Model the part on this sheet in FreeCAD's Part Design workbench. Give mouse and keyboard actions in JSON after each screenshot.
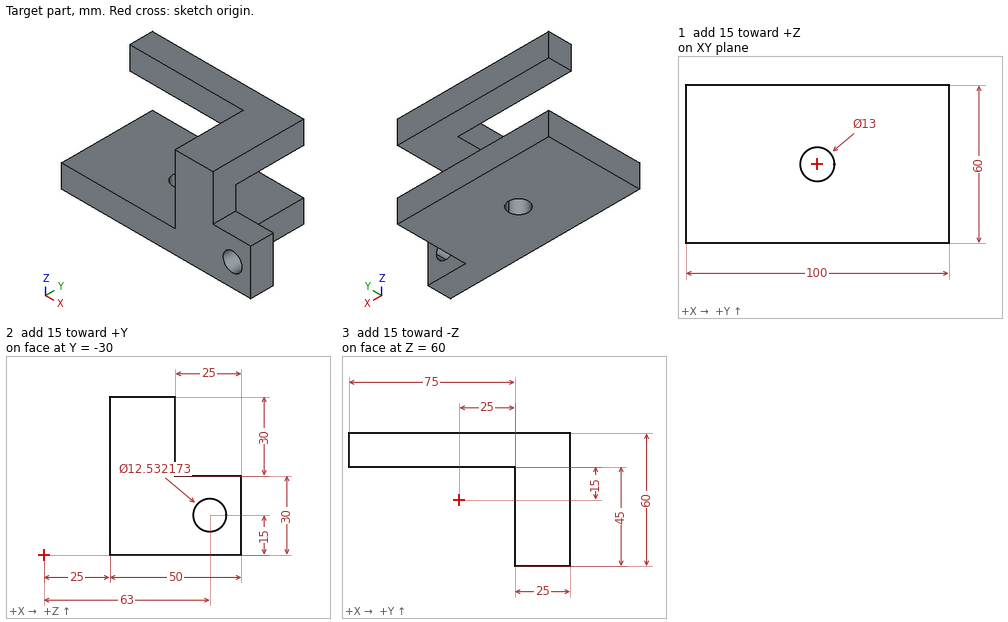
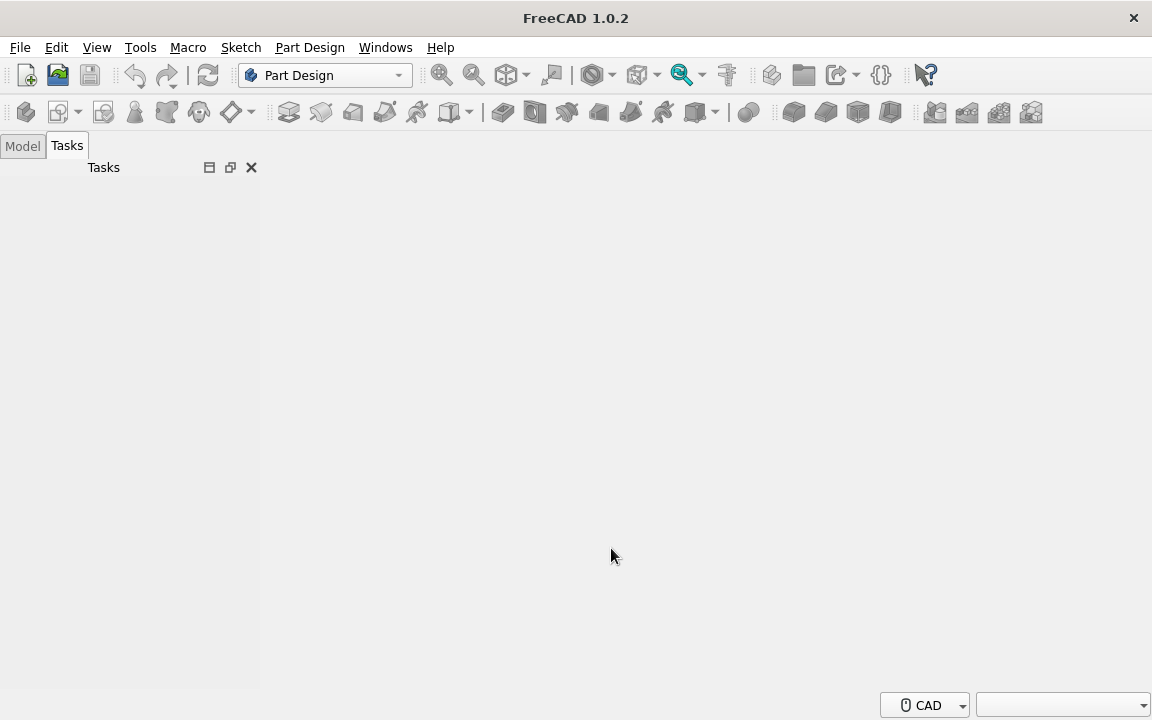
{"action": "key", "text": "ctrl+n"}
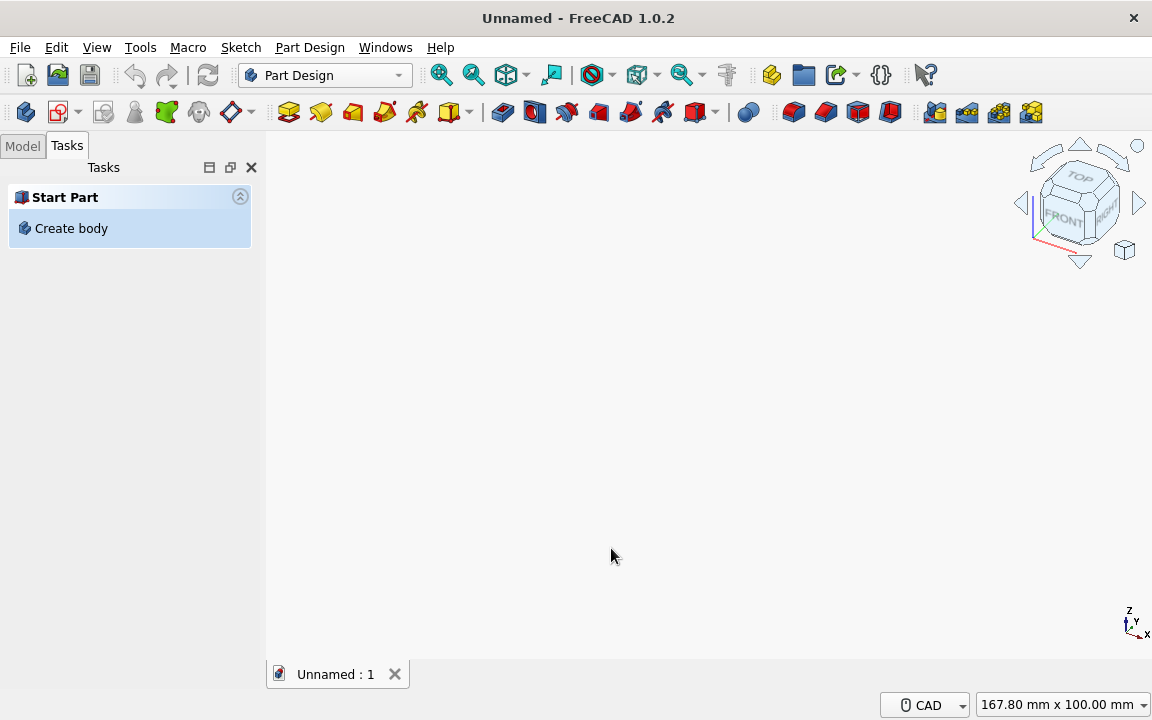
{"action": "left_click", "coordinate": [58, 112]}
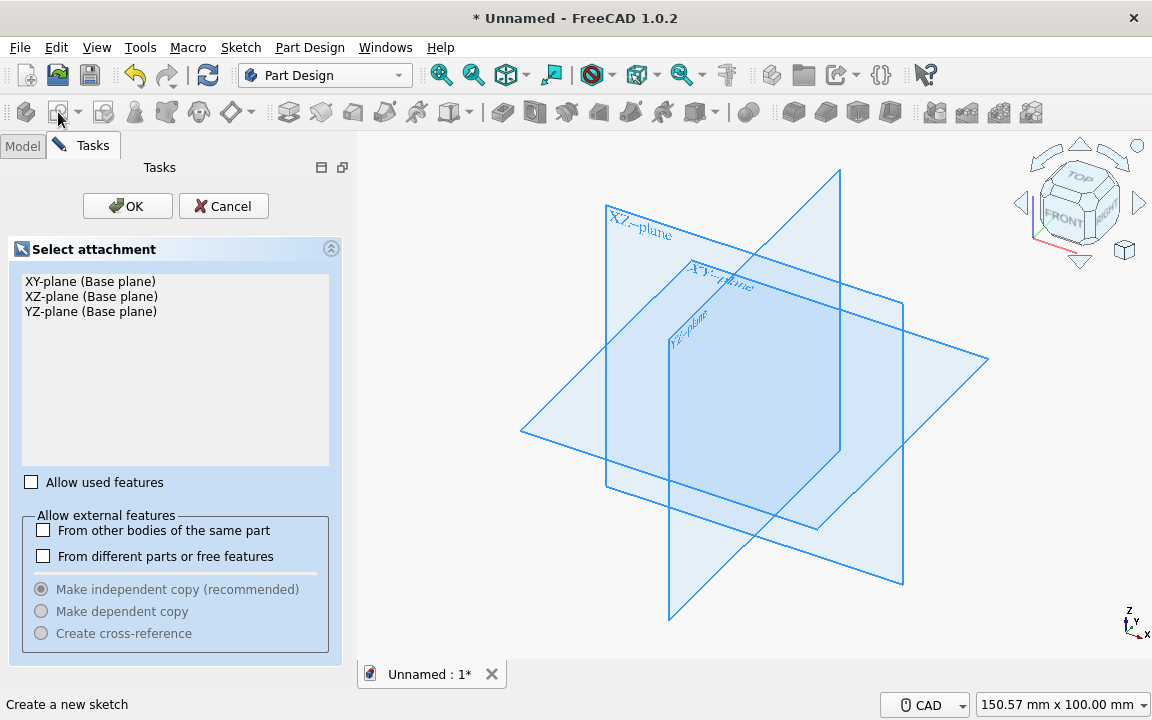
{"action": "left_click", "coordinate": [82, 282]}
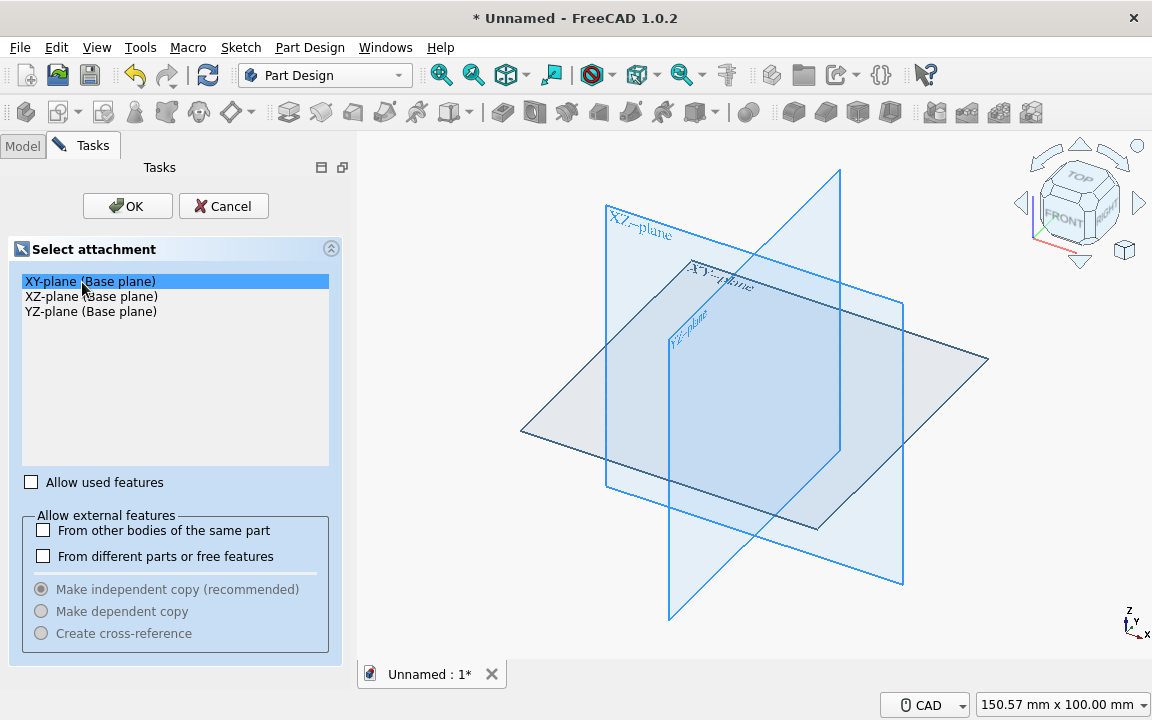
{"action": "left_click", "coordinate": [128, 206]}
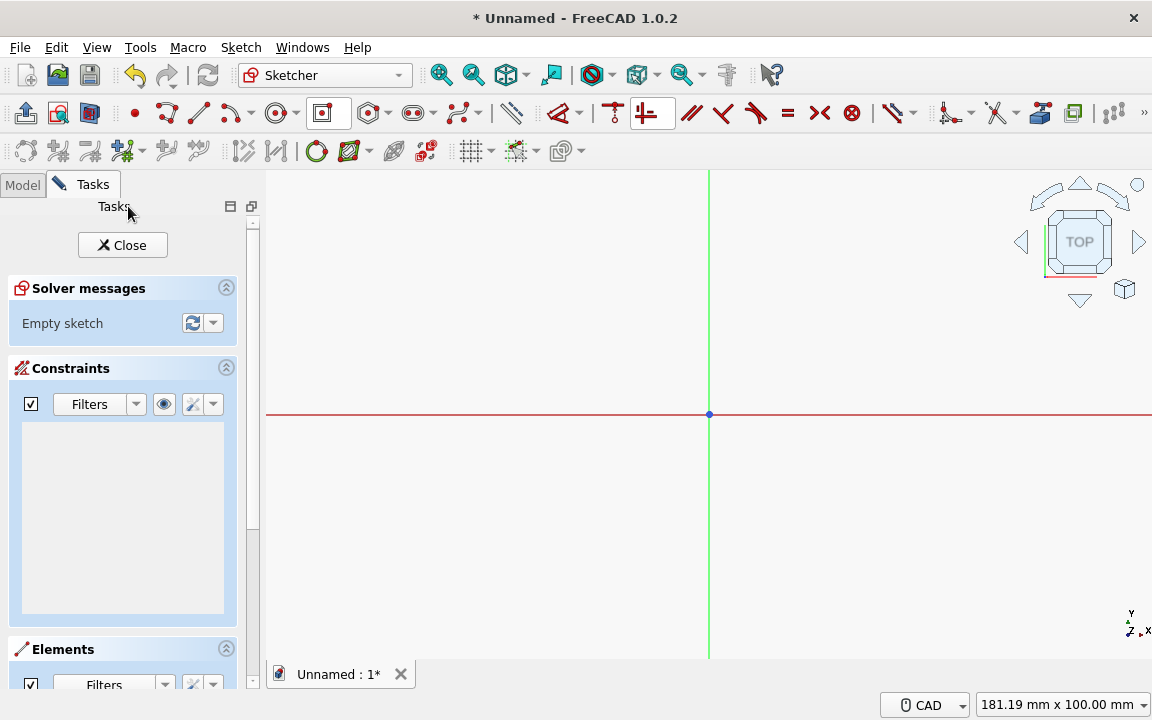
{"action": "key", "text": "g v"}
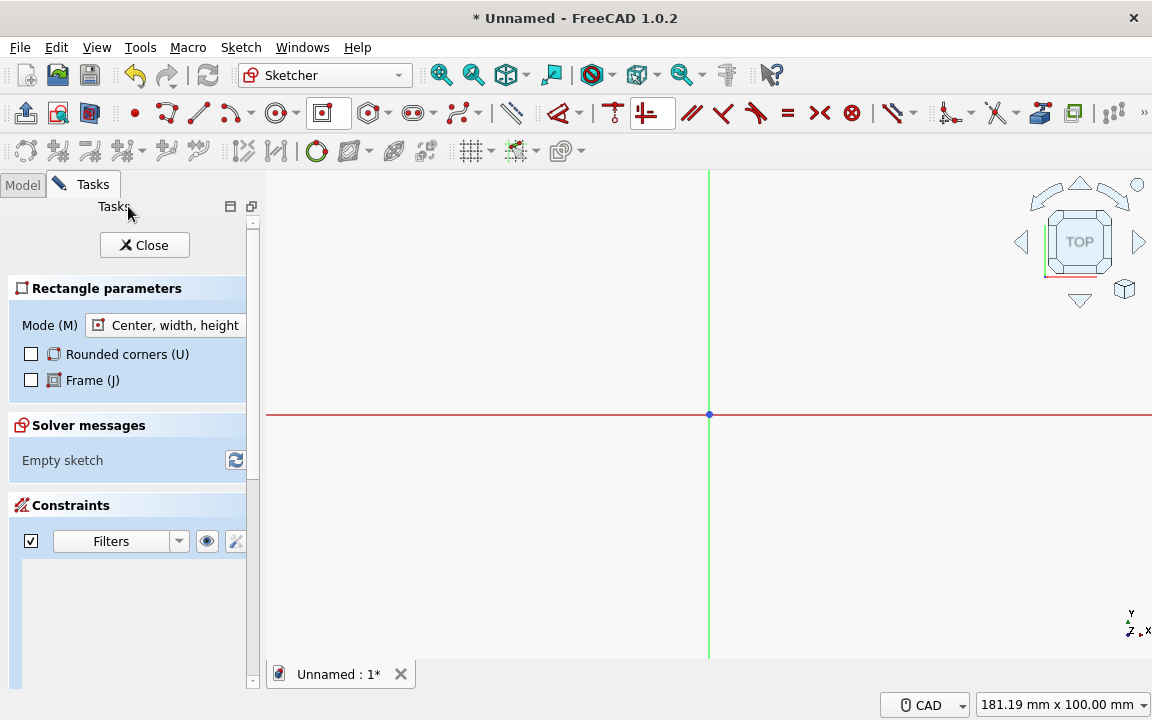
{"action": "left_click", "coordinate": [709, 414]}
{"action": "left_click", "coordinate": [954, 268]}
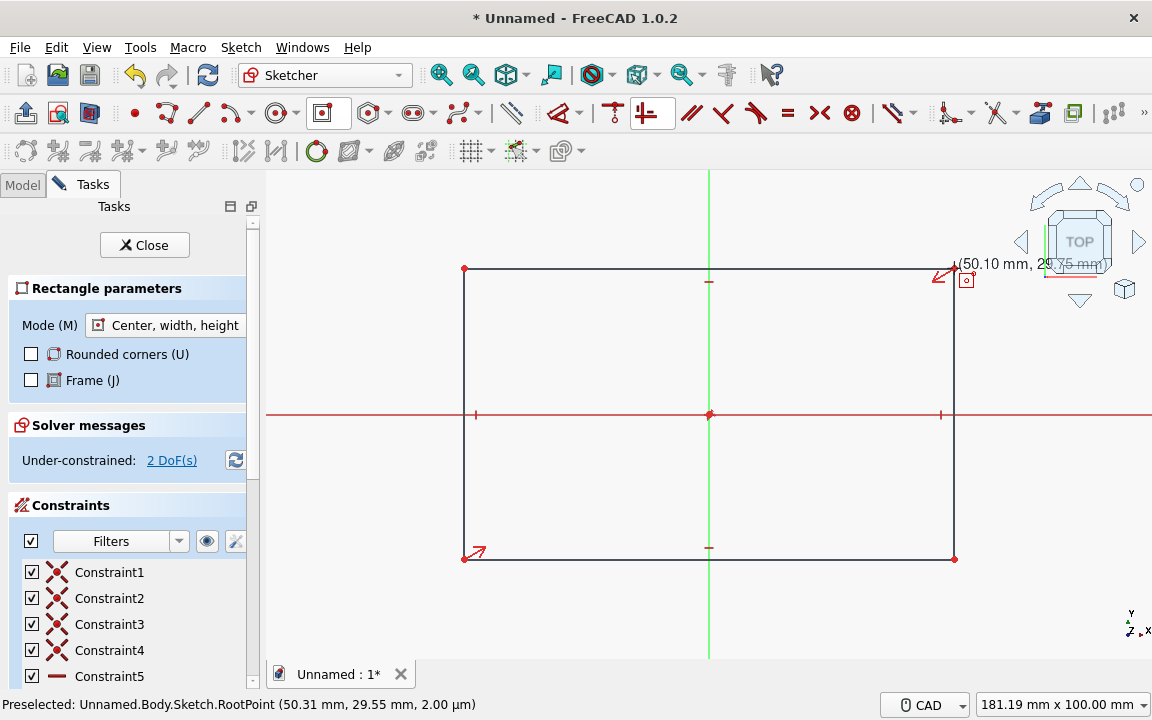
{"action": "key", "text": "g c"}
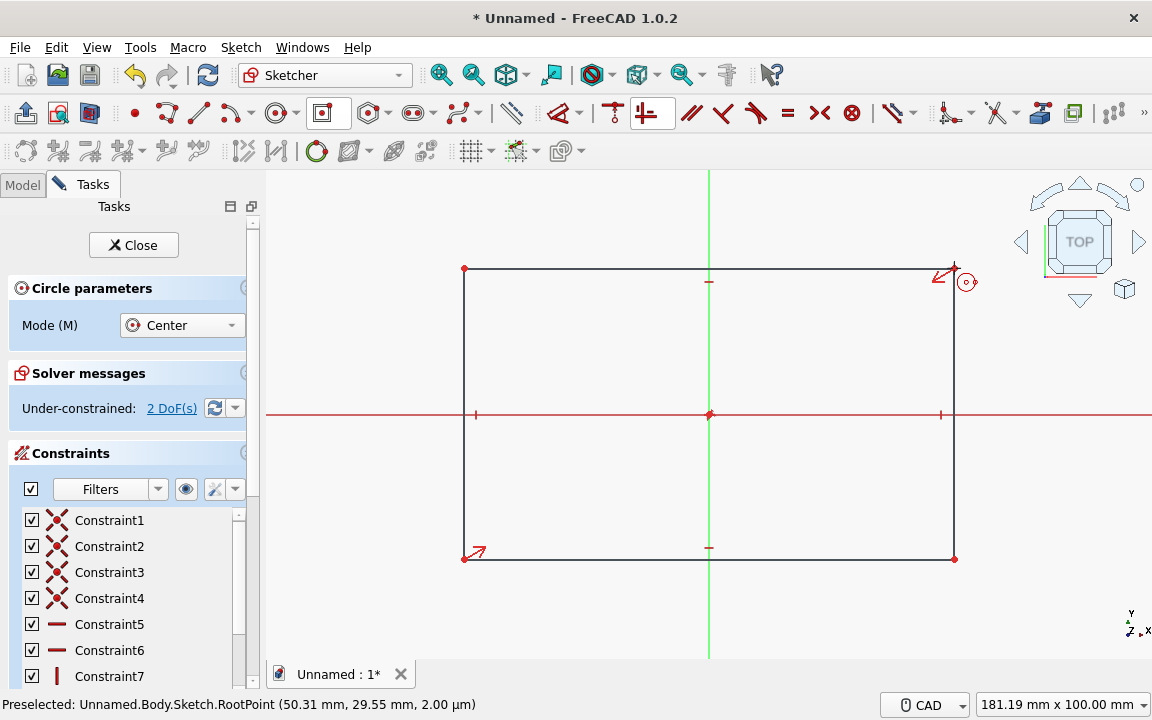
{"action": "left_click", "coordinate": [709, 414]}
{"action": "left_click", "coordinate": [731, 392]}
{"action": "key", "text": "Escape"}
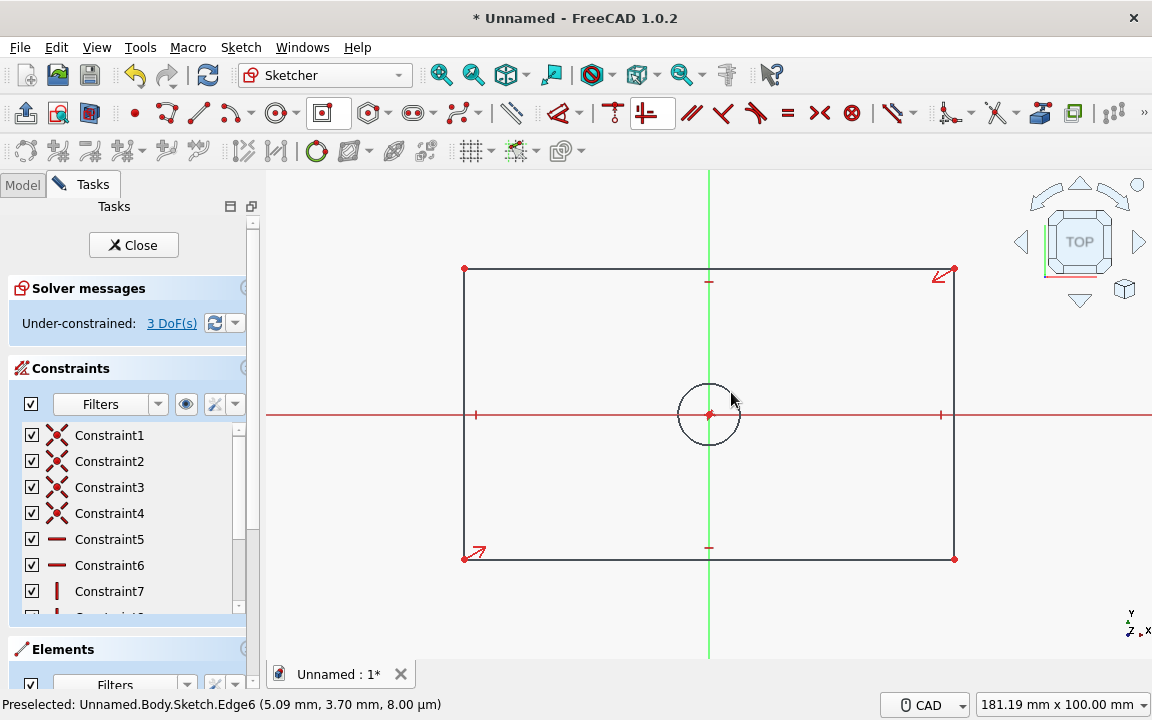
{"action": "key", "text": "d"}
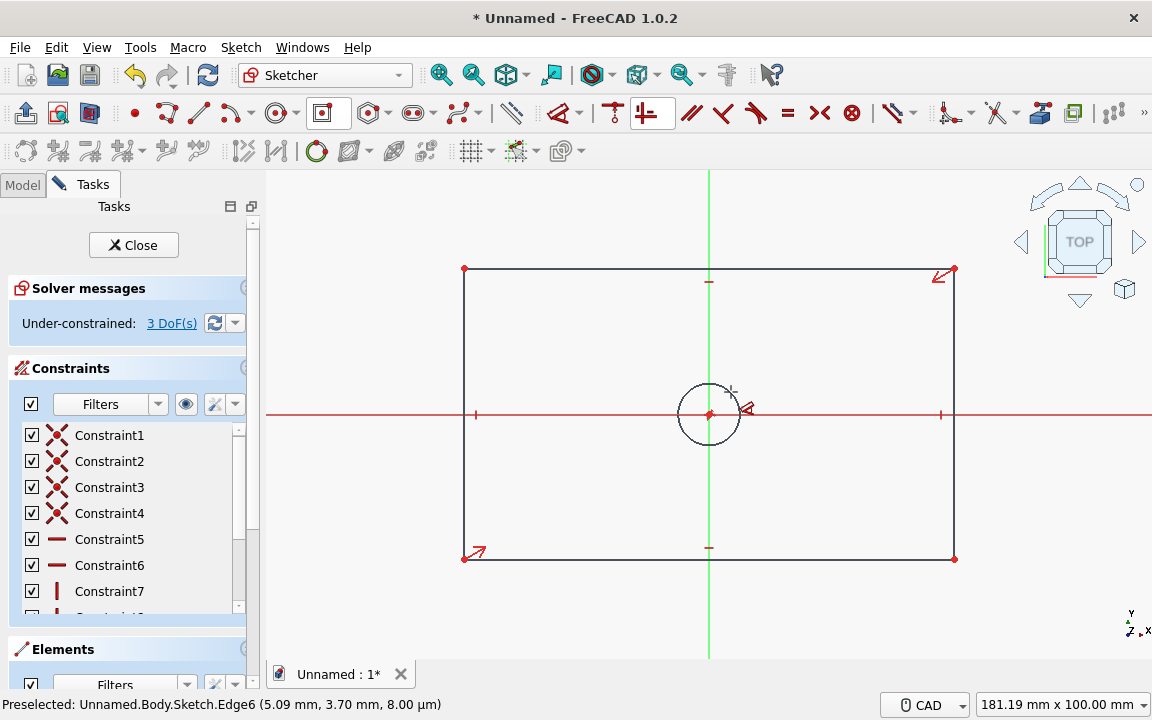
{"action": "left_click", "coordinate": [731, 393]}
{"action": "left_click", "coordinate": [754, 371]}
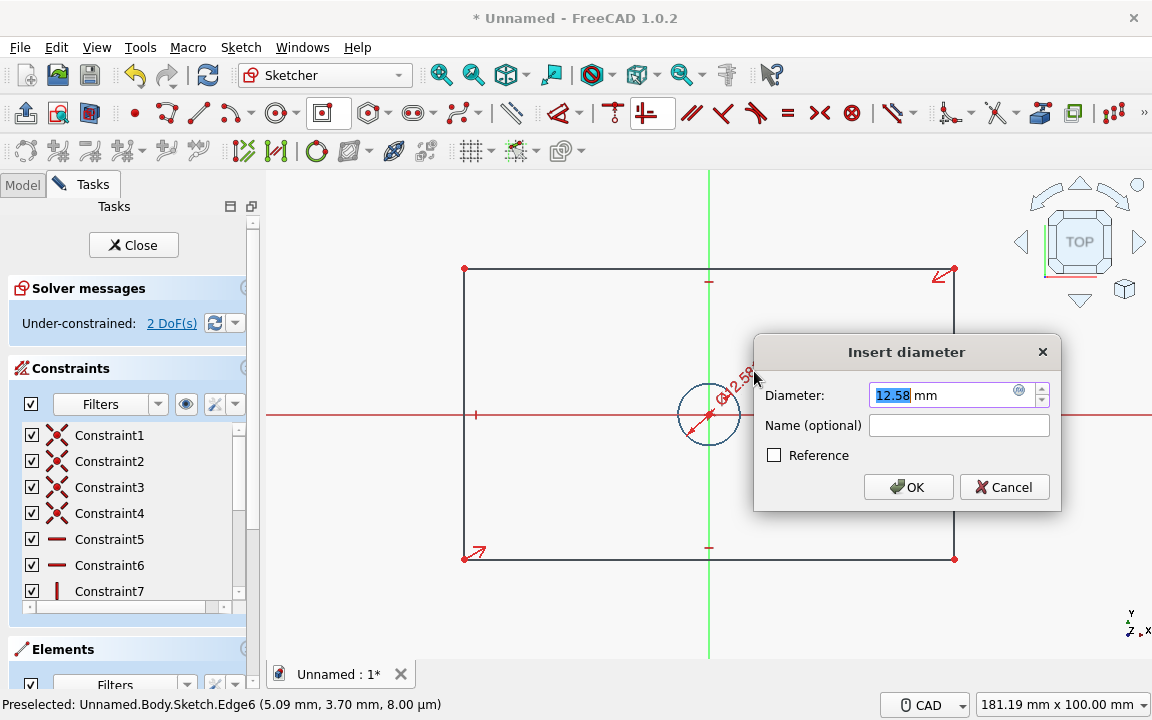
{"action": "type", "text": "13"}
{"action": "key", "text": "Return"}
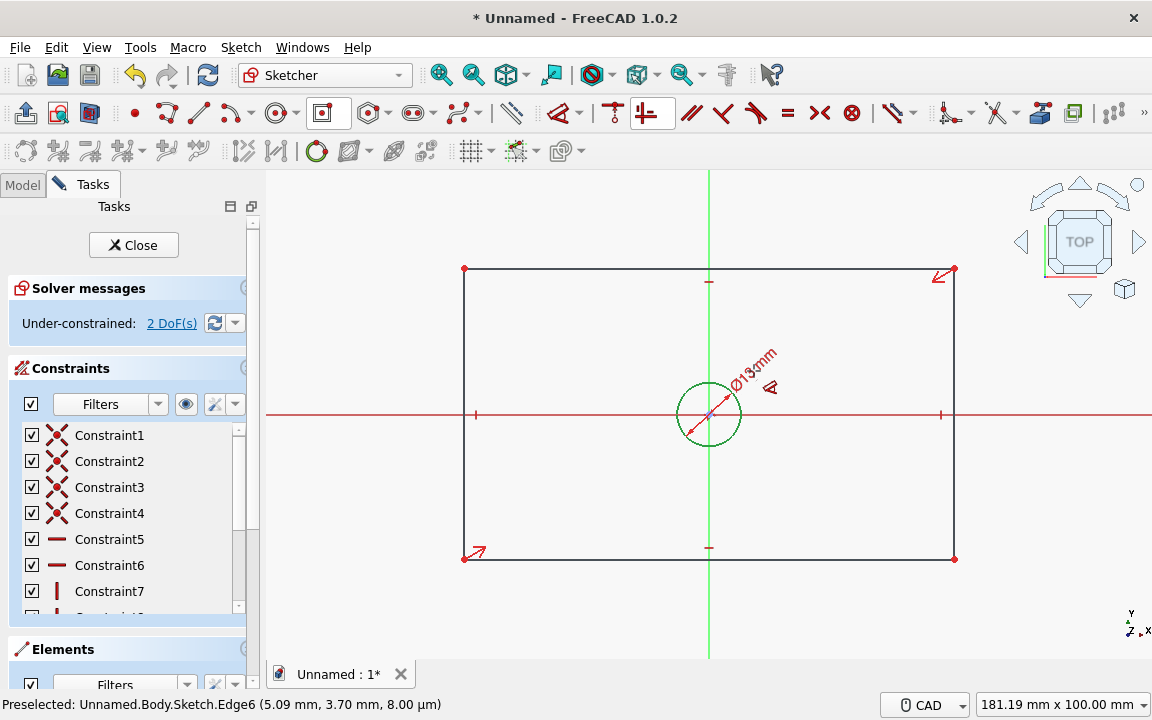
{"action": "left_click", "coordinate": [954, 473]}
{"action": "left_click", "coordinate": [920, 348]}